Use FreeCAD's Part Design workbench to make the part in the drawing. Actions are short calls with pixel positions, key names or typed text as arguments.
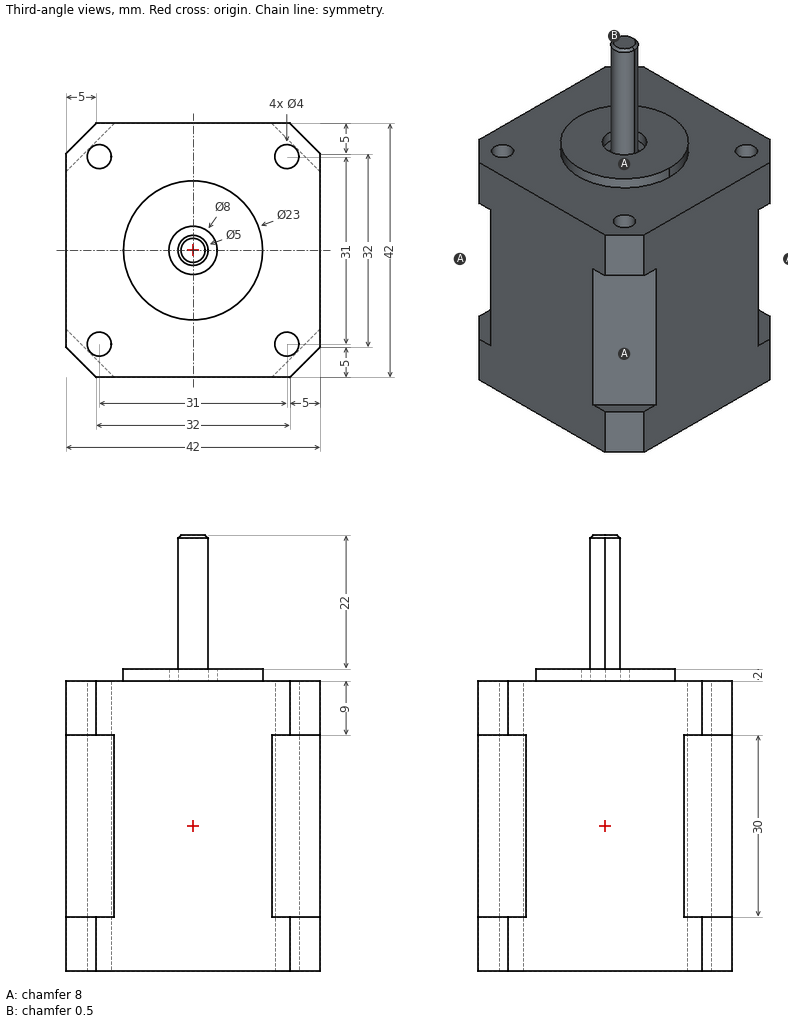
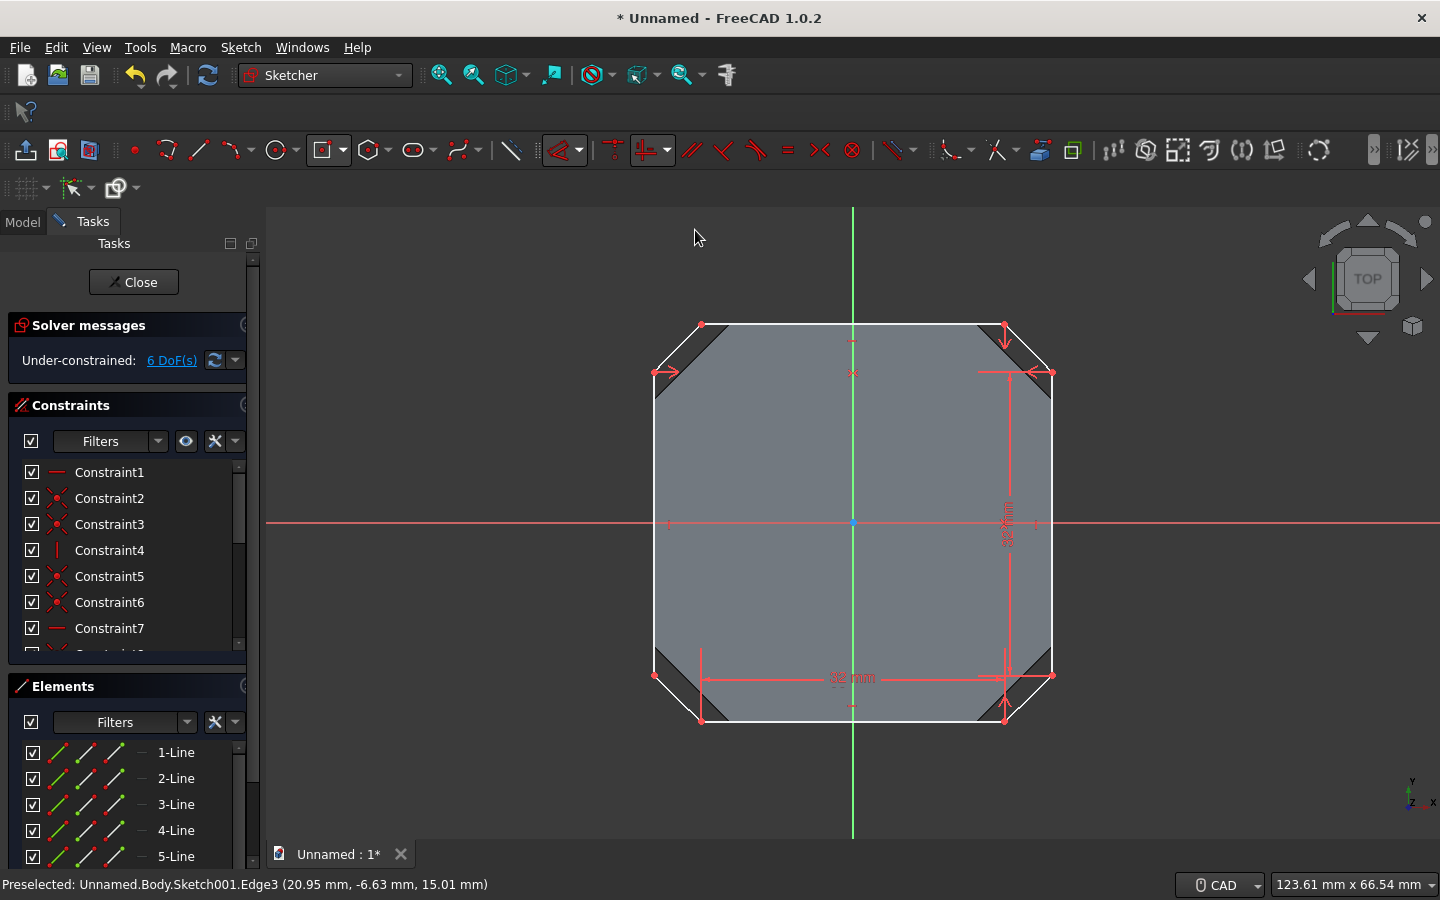
click(914, 324)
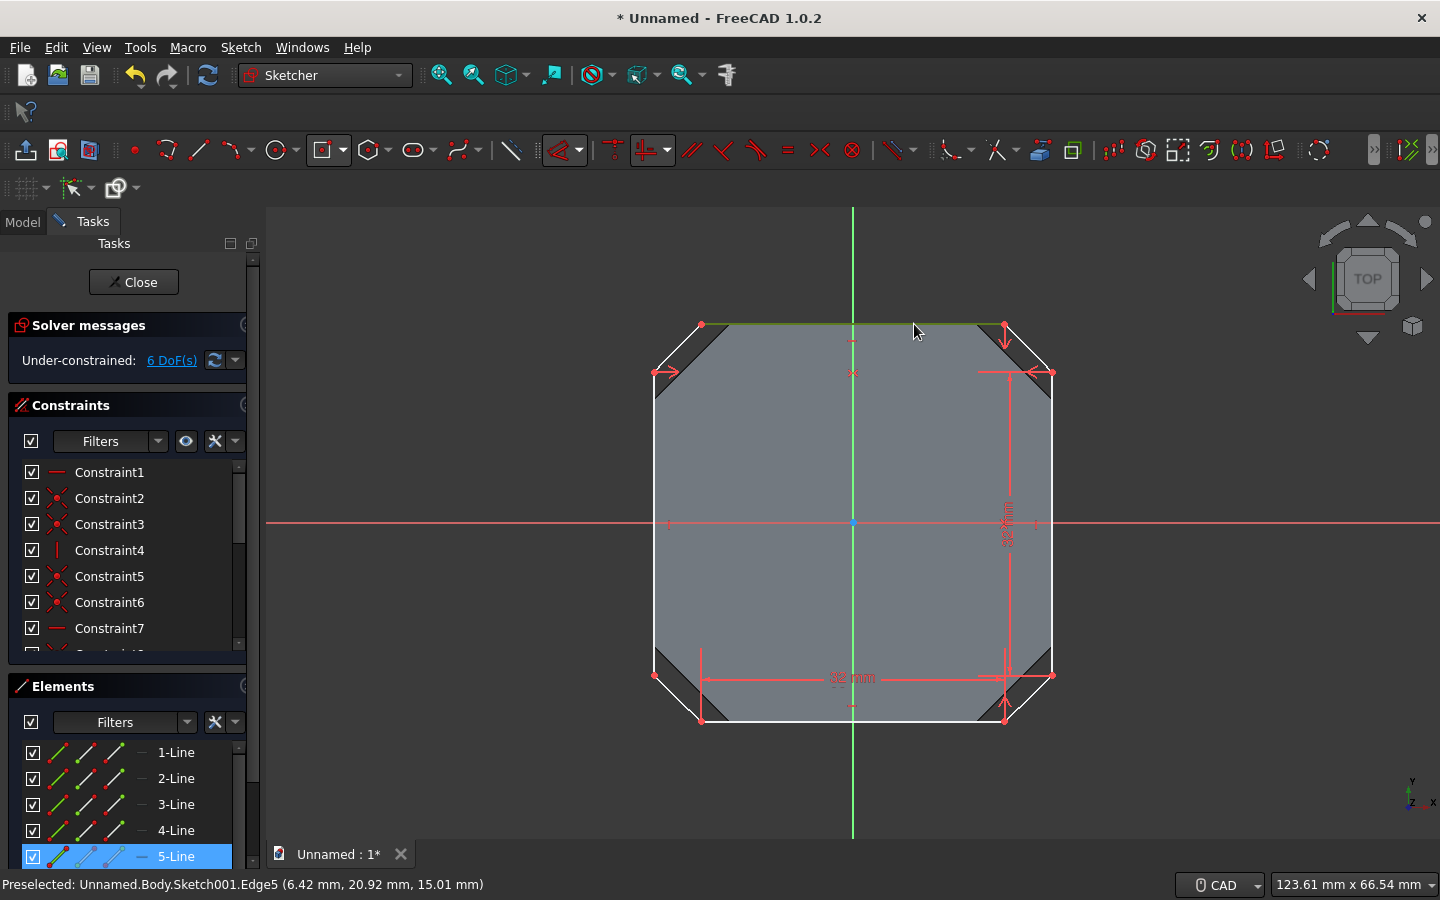
key(l)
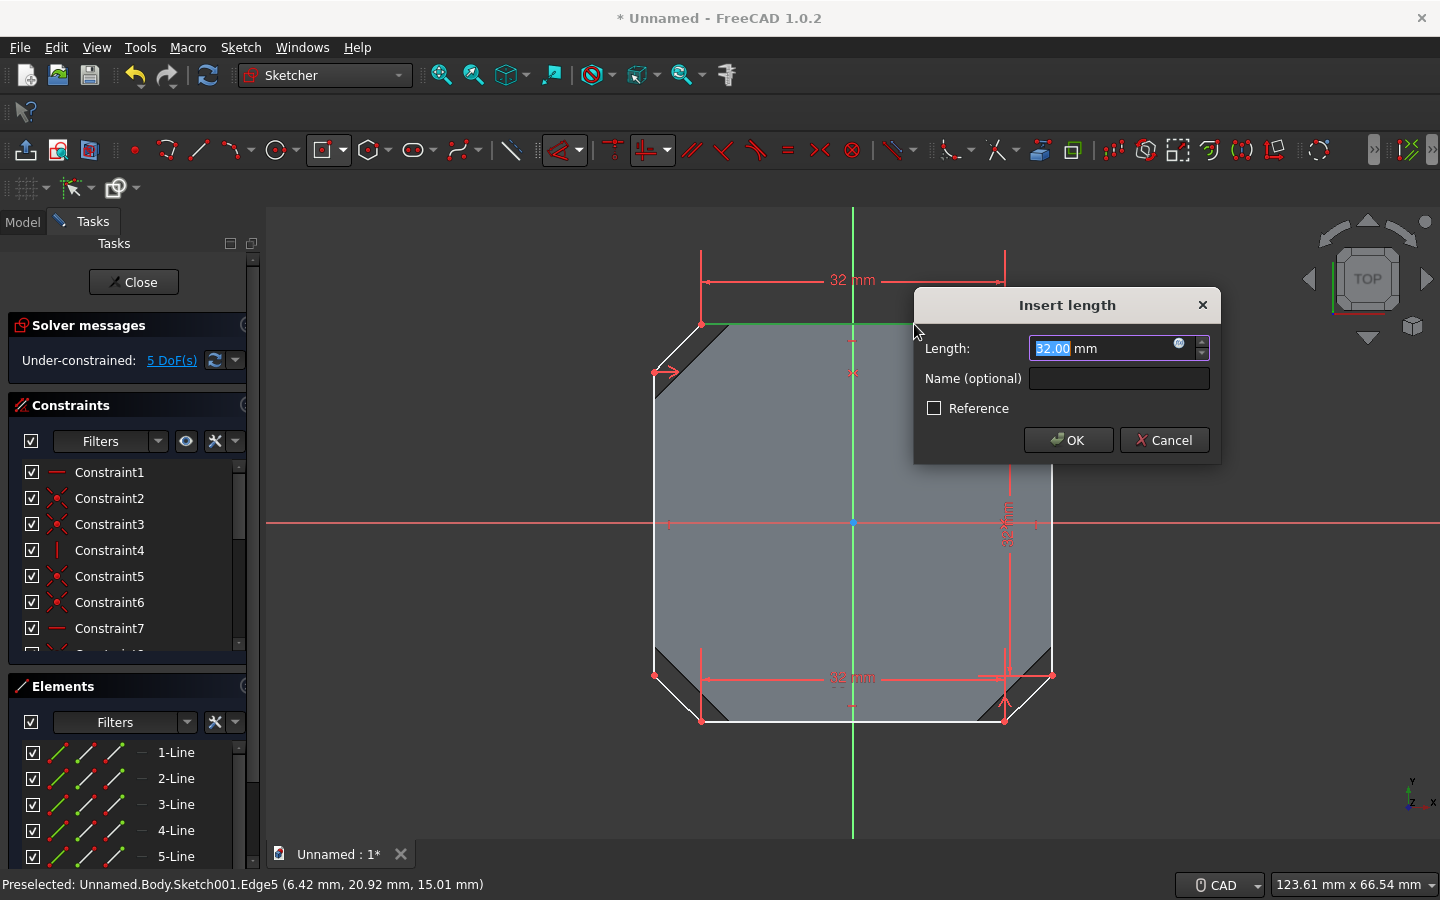
text(32)
key(Return)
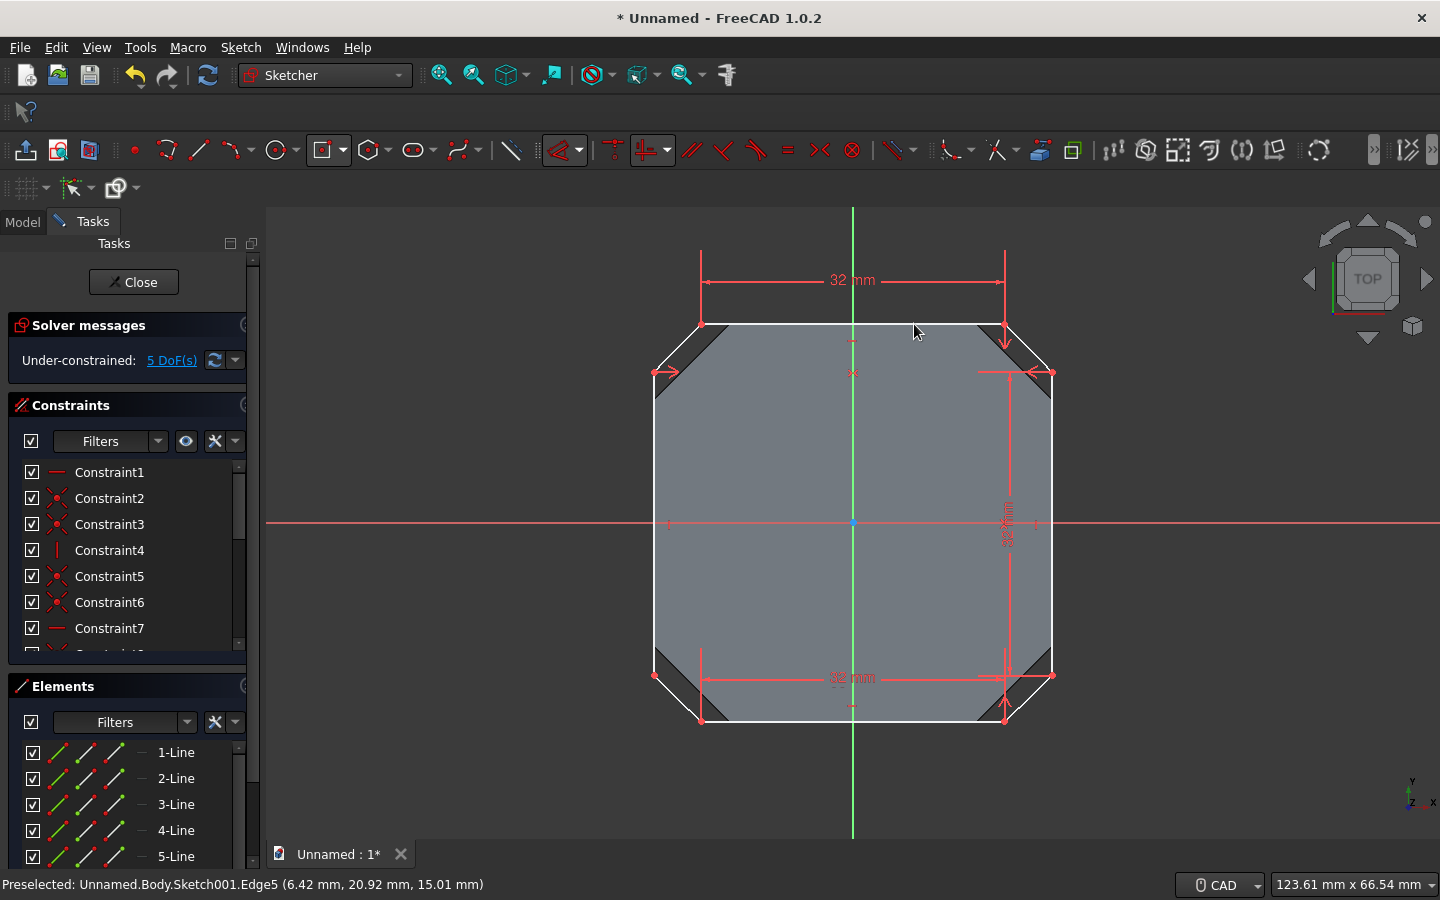
click(654, 463)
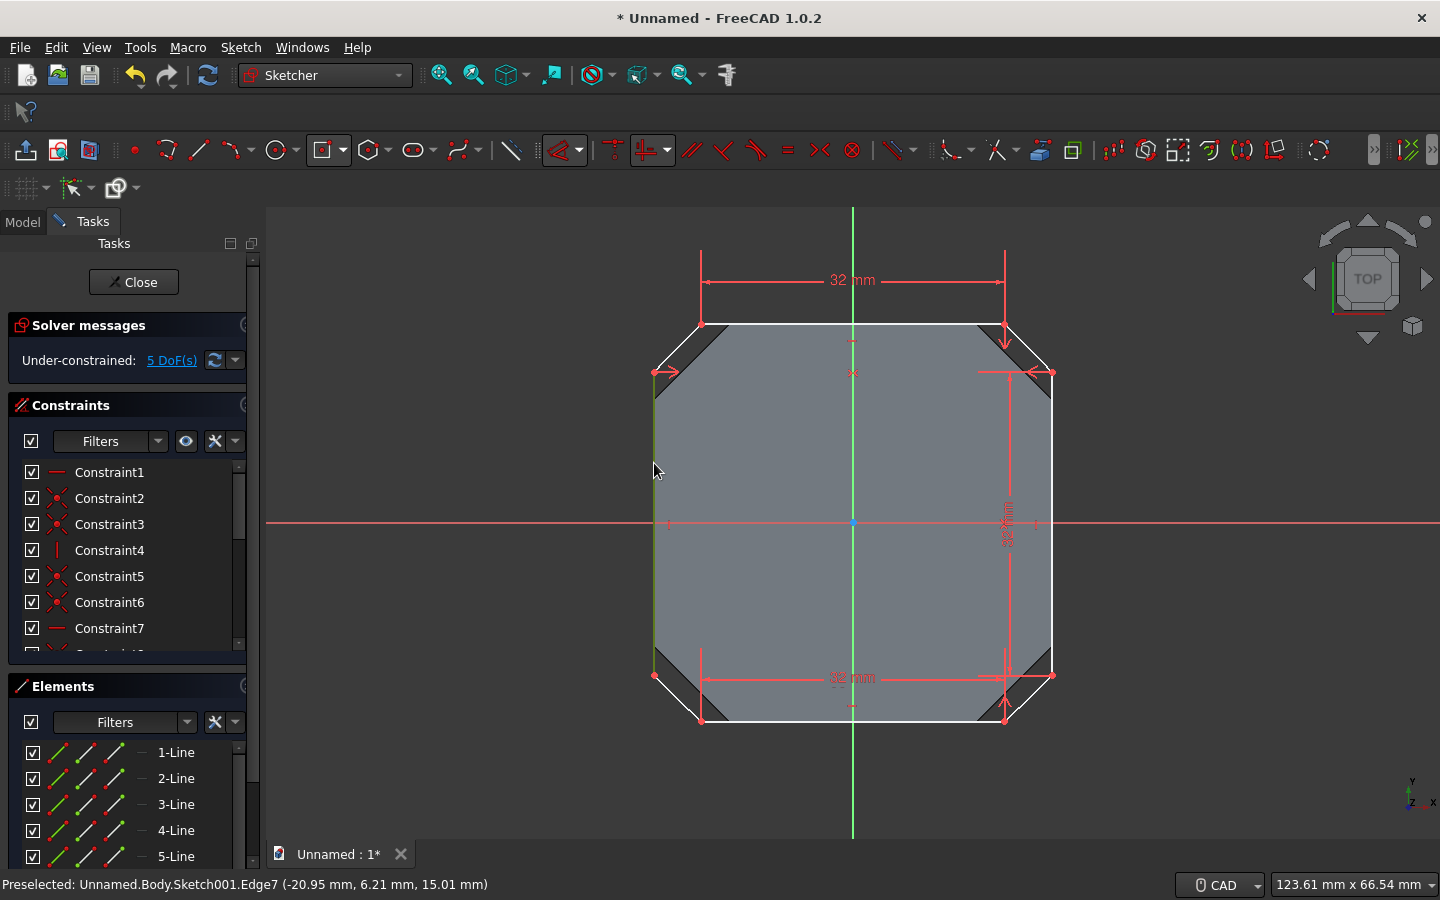
click(582, 150)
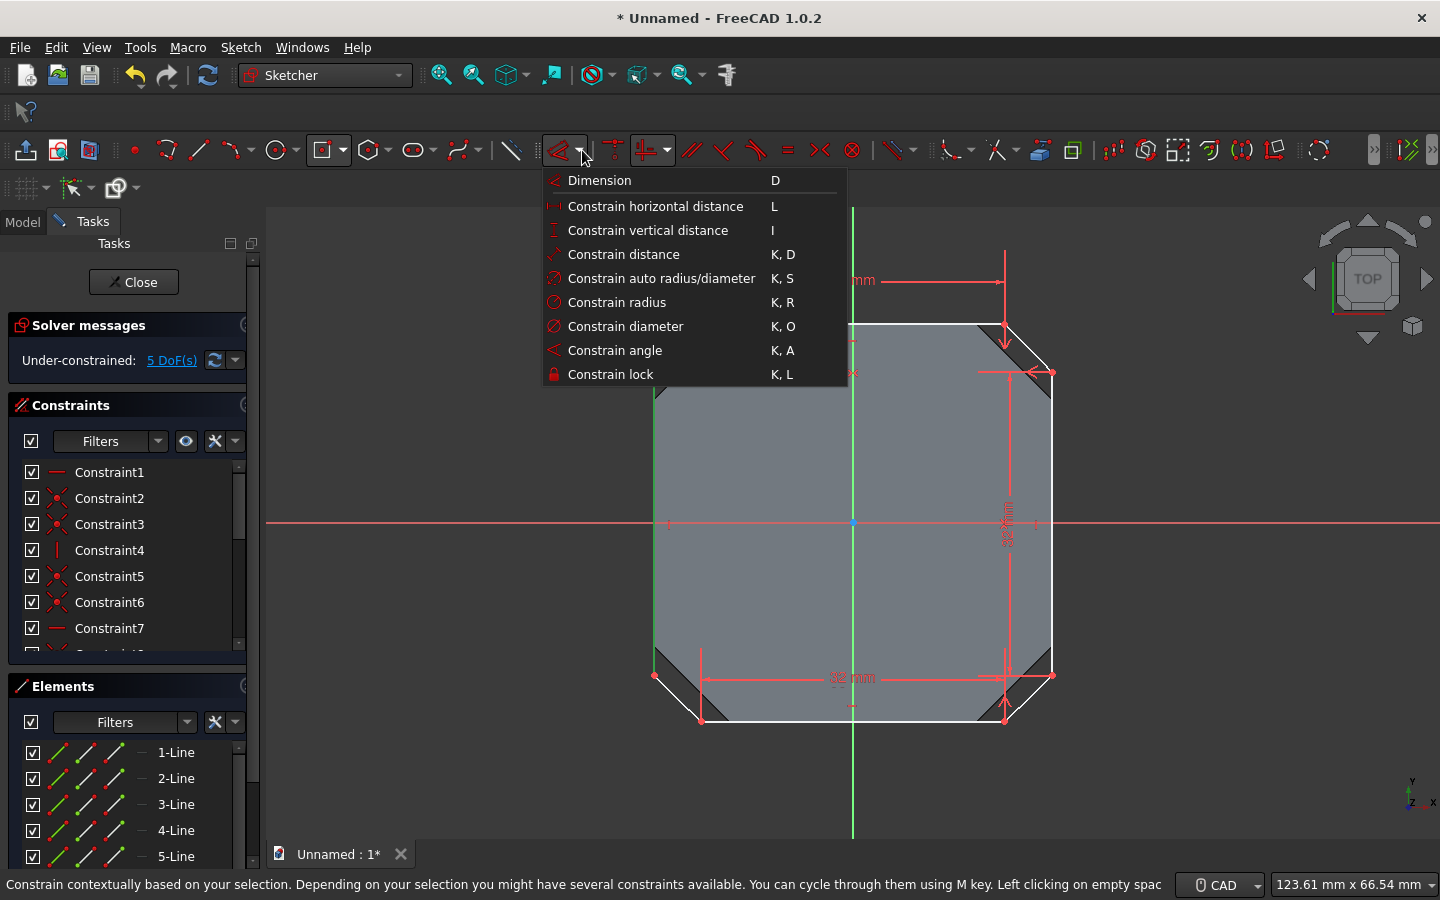
click(695, 230)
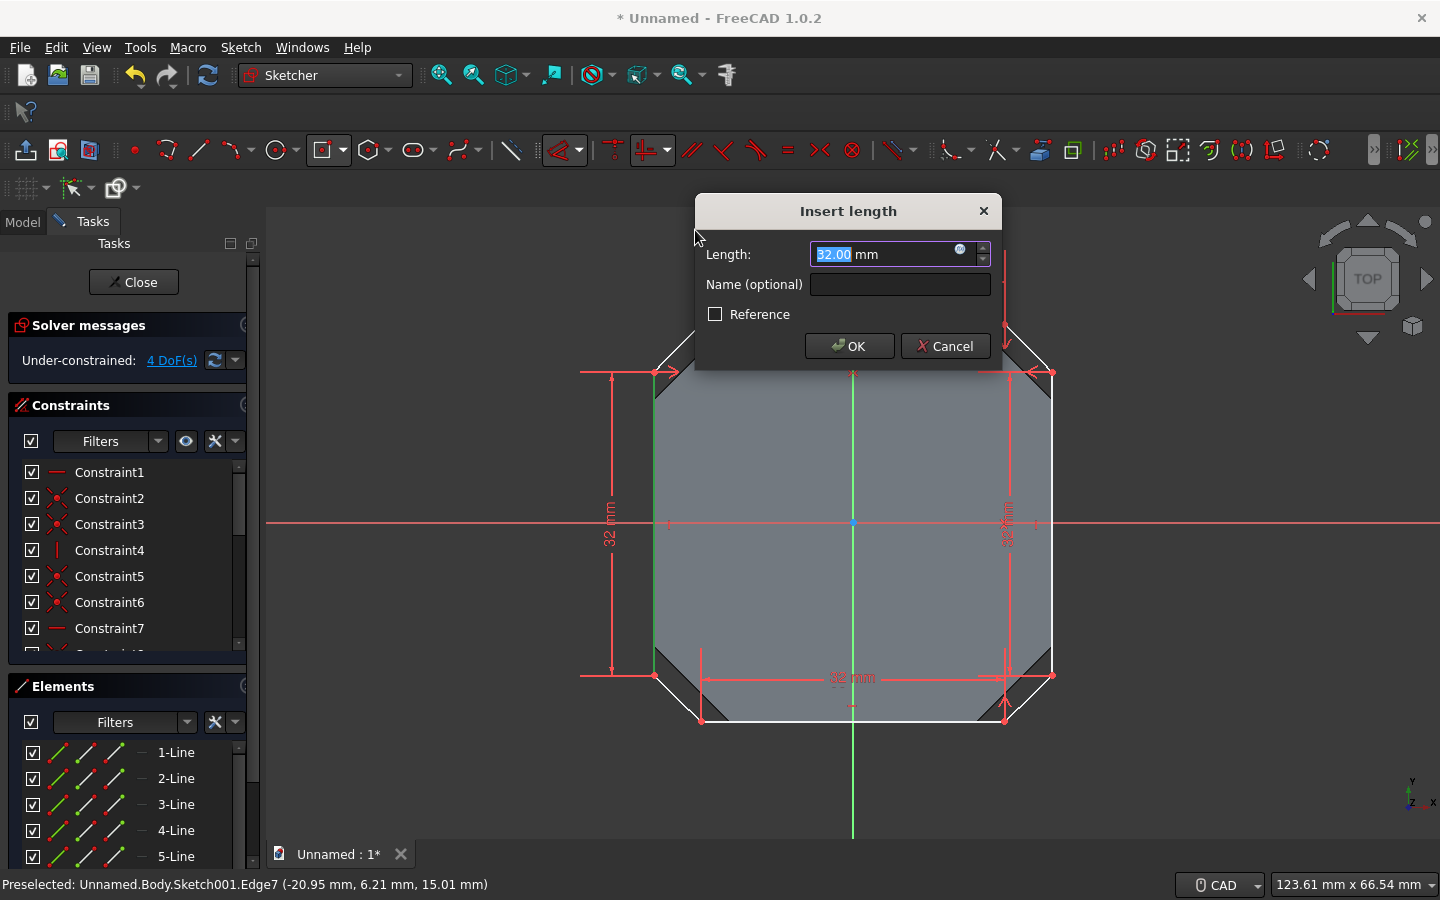
text(32)
key(Return)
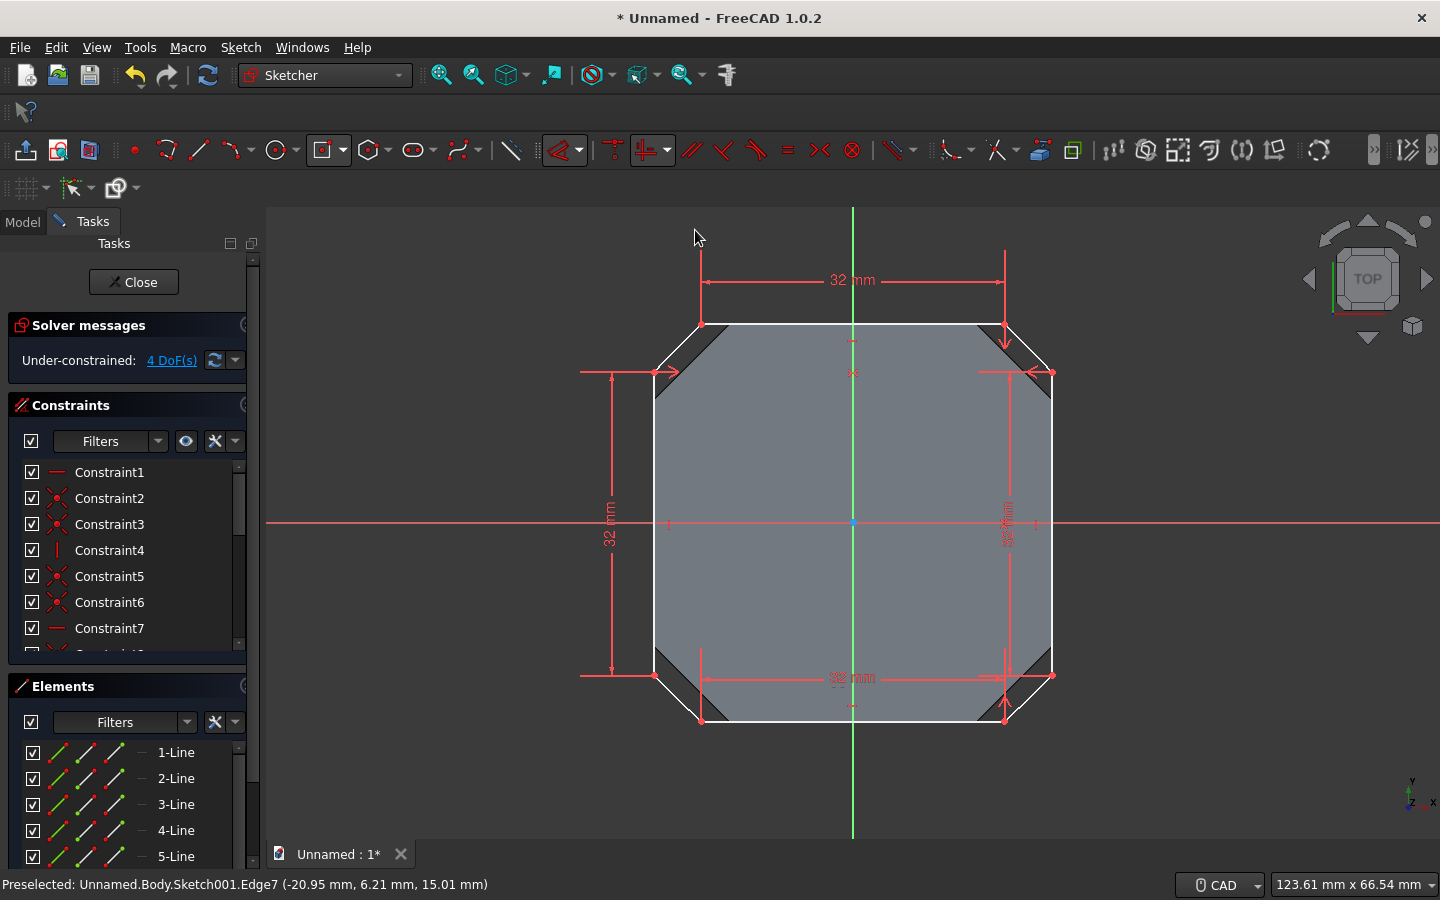
click(1019, 708)